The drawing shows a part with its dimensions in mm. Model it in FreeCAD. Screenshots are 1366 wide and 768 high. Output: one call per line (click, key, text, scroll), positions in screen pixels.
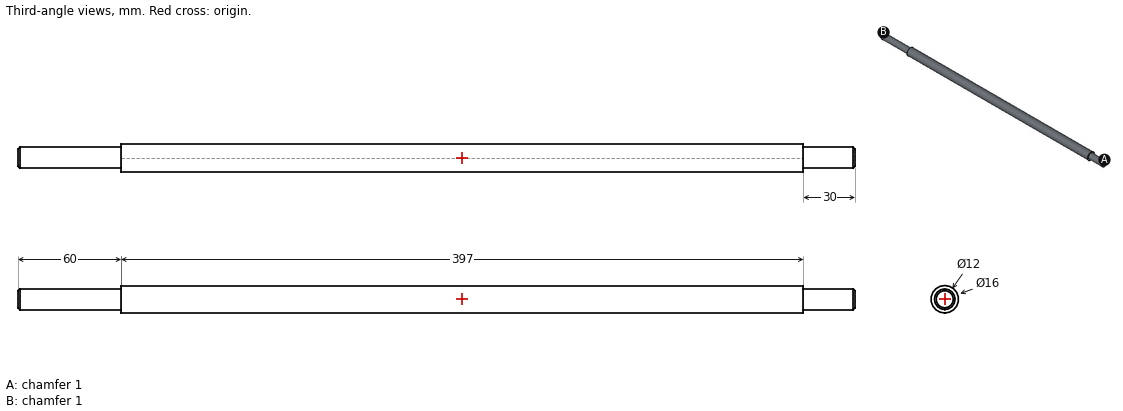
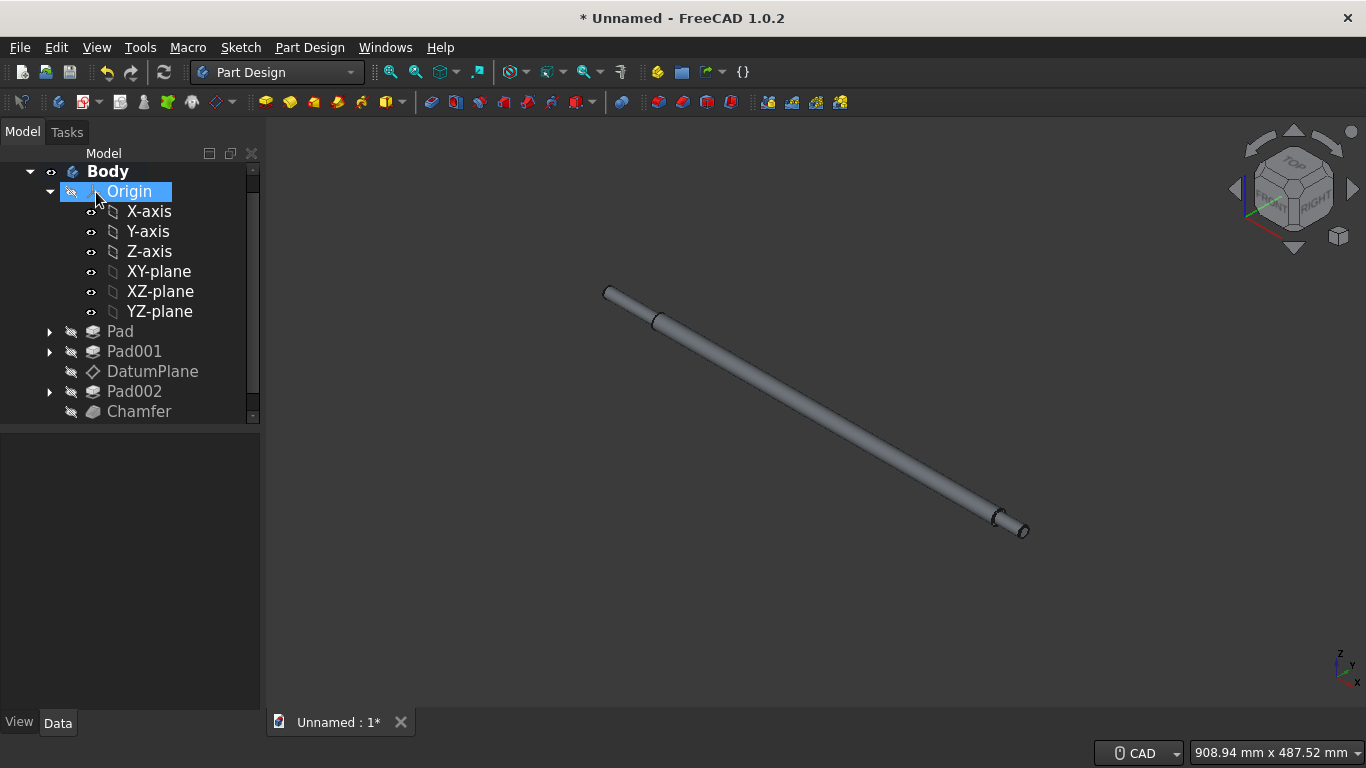
key(v)
key(f)